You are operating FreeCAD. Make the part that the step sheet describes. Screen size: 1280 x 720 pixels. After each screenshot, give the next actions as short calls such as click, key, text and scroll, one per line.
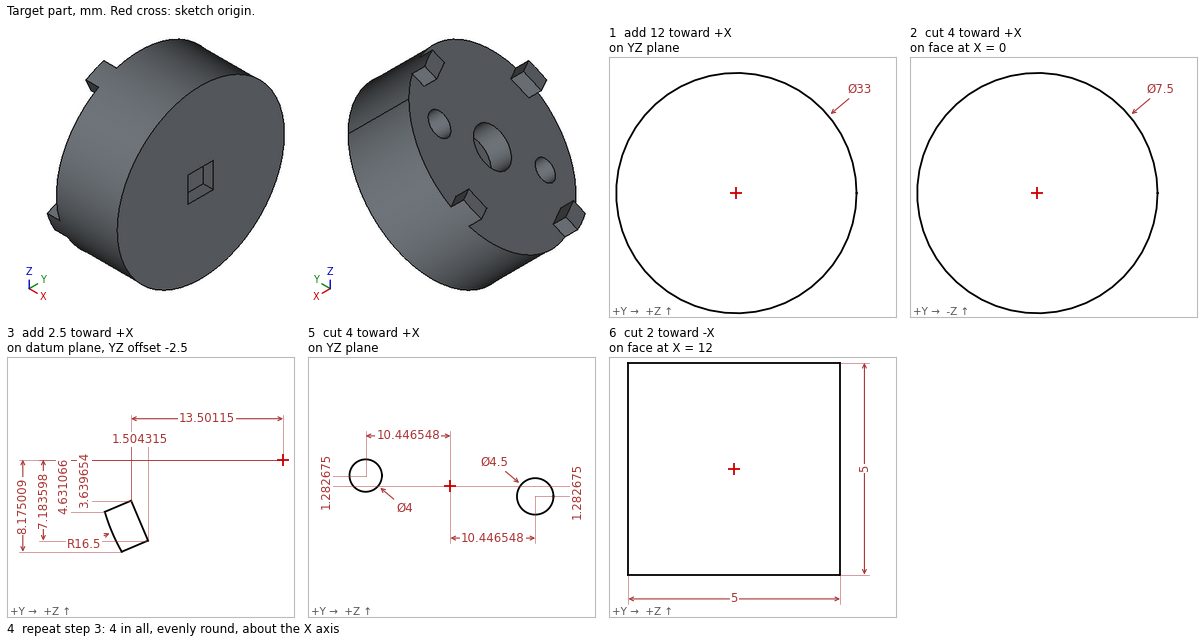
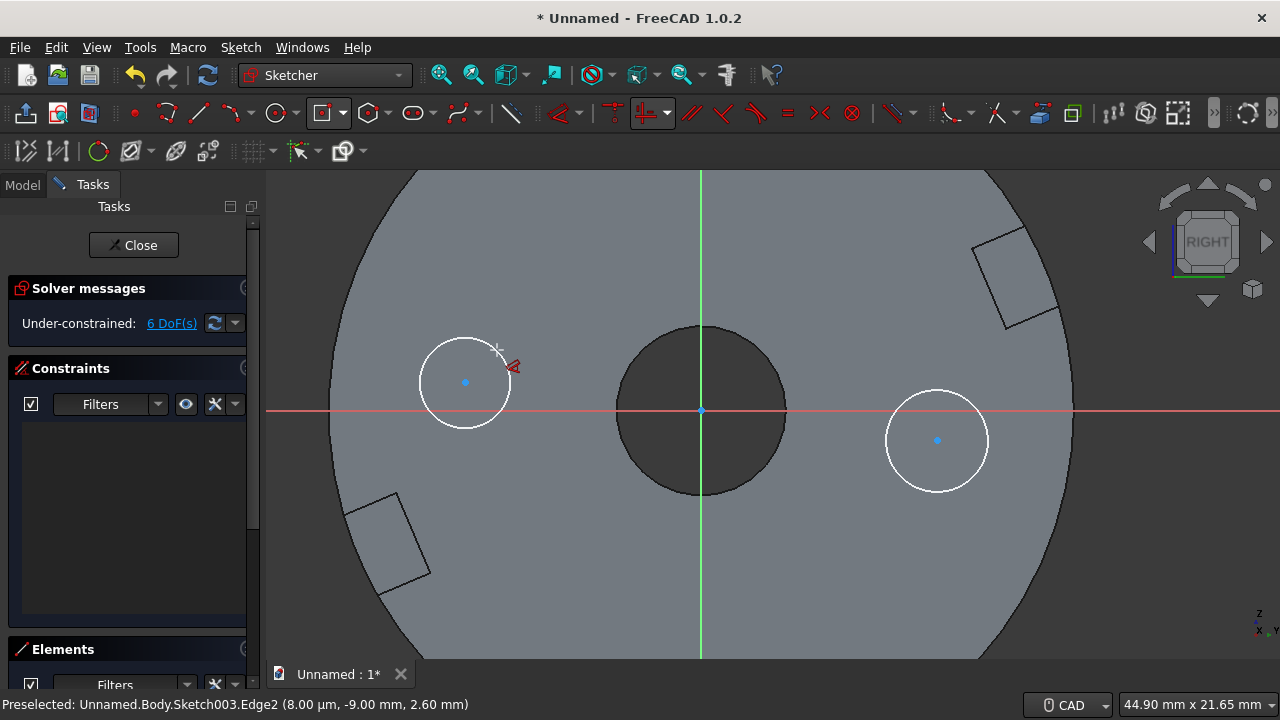
click(901, 477)
click(878, 500)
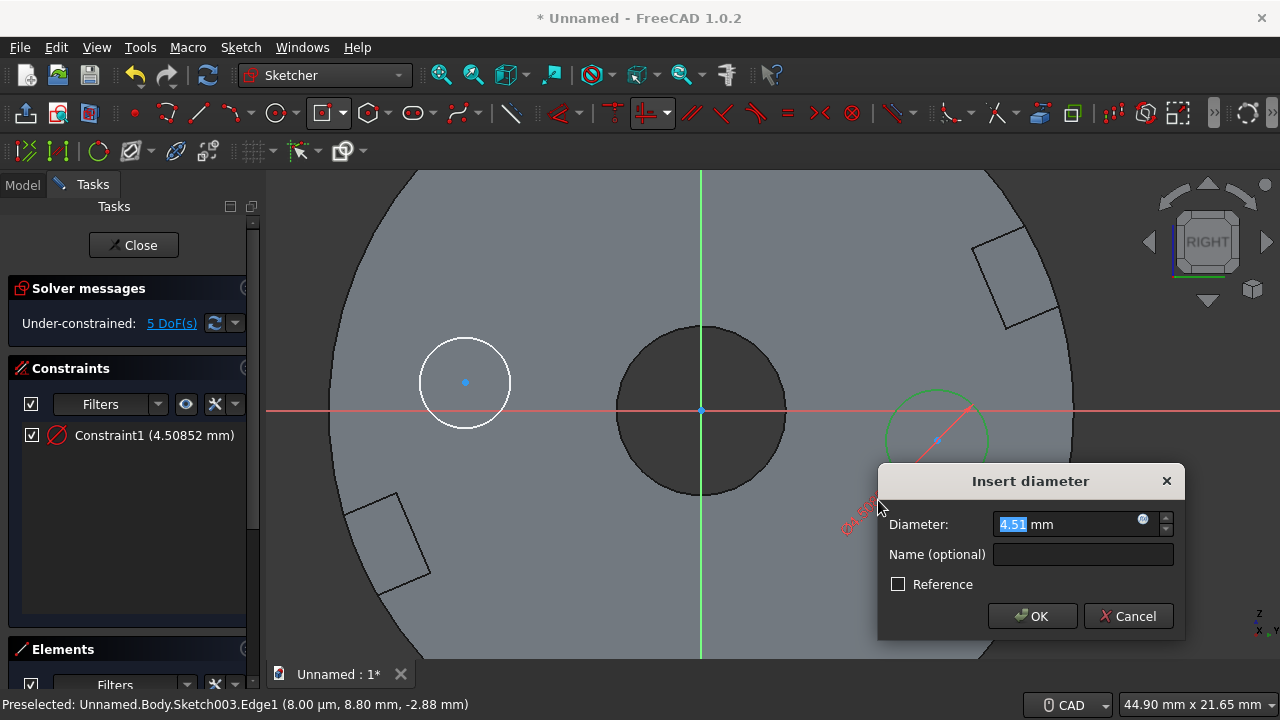
text(4.5)
key(Return)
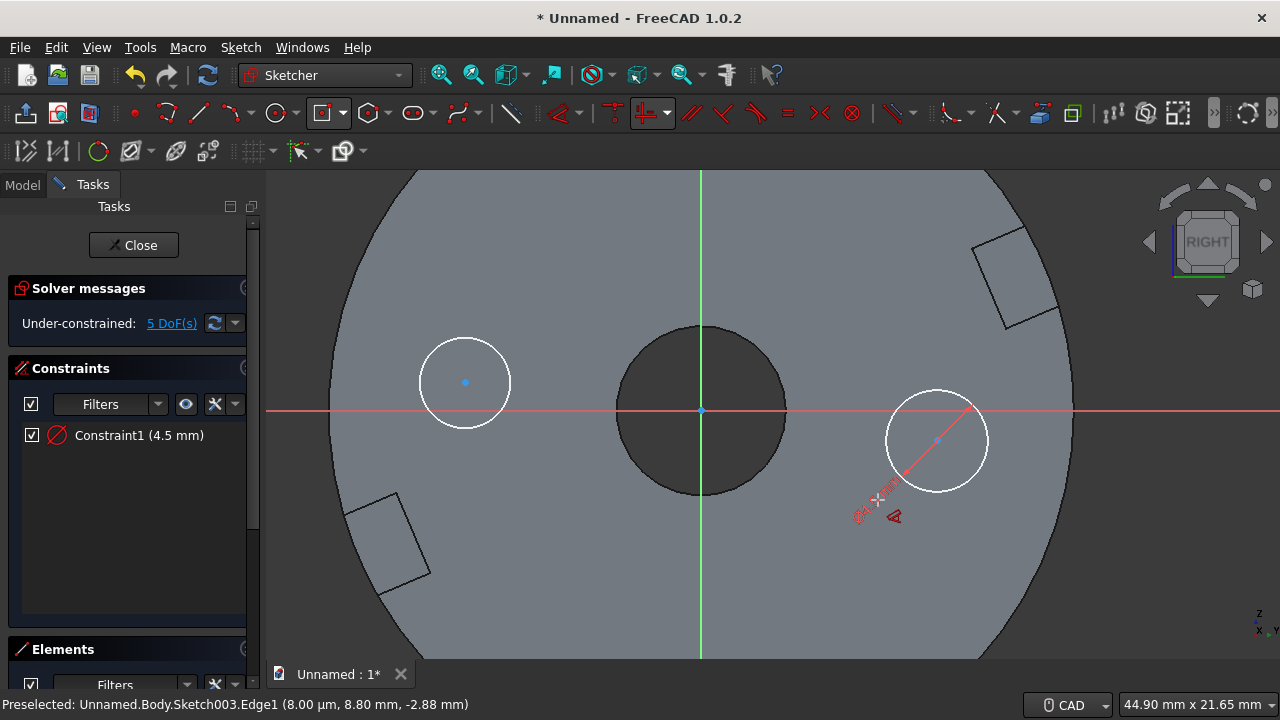
click(497, 351)
click(520, 328)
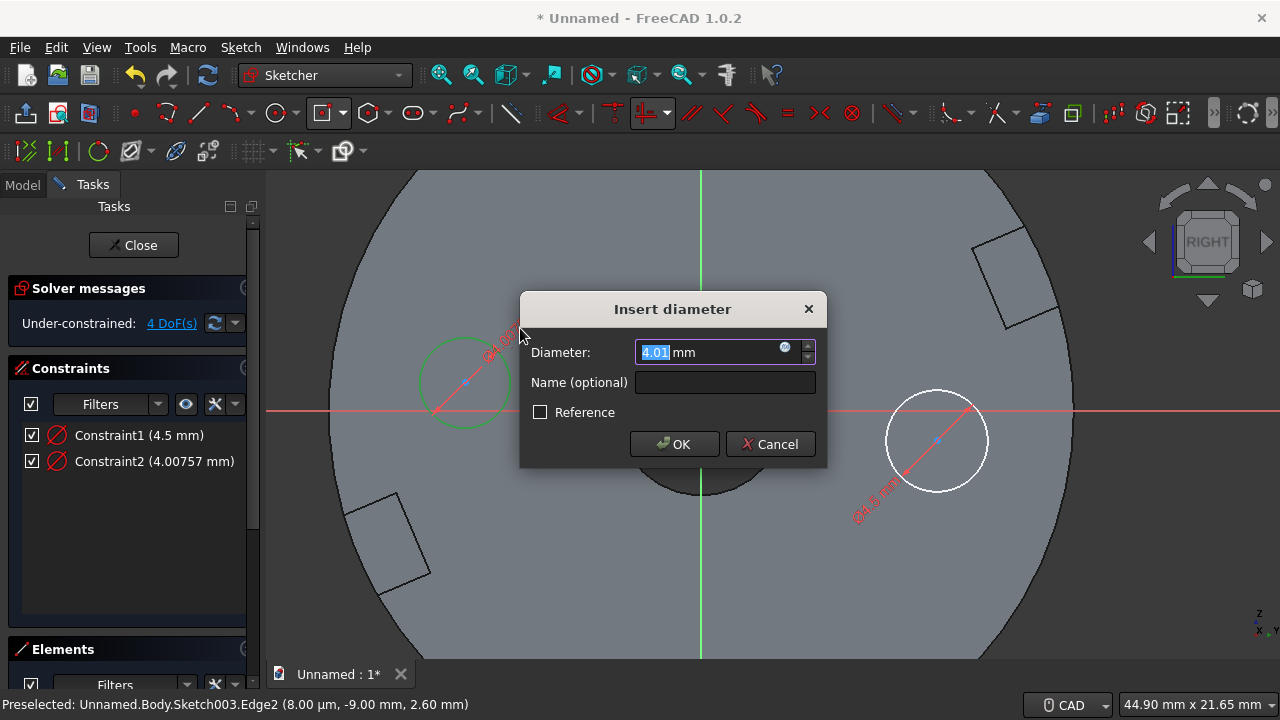
text(4)
key(Return)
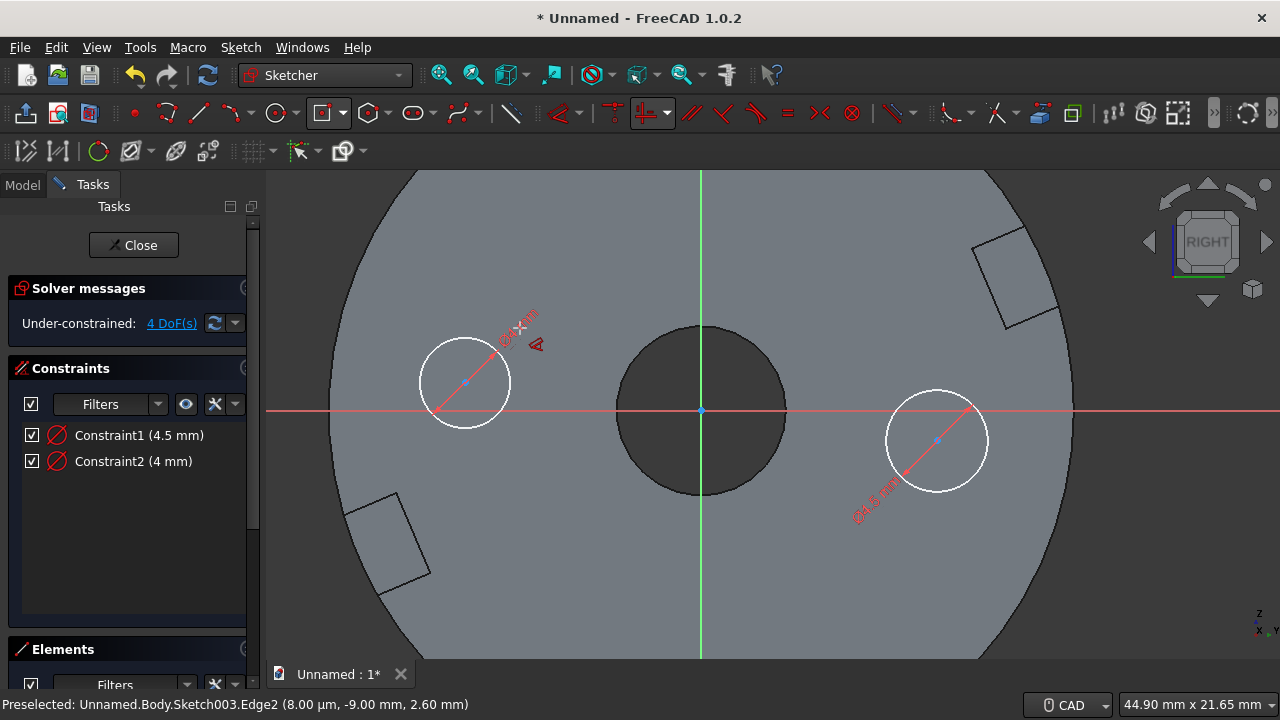
scroll(937, 441, up, 2)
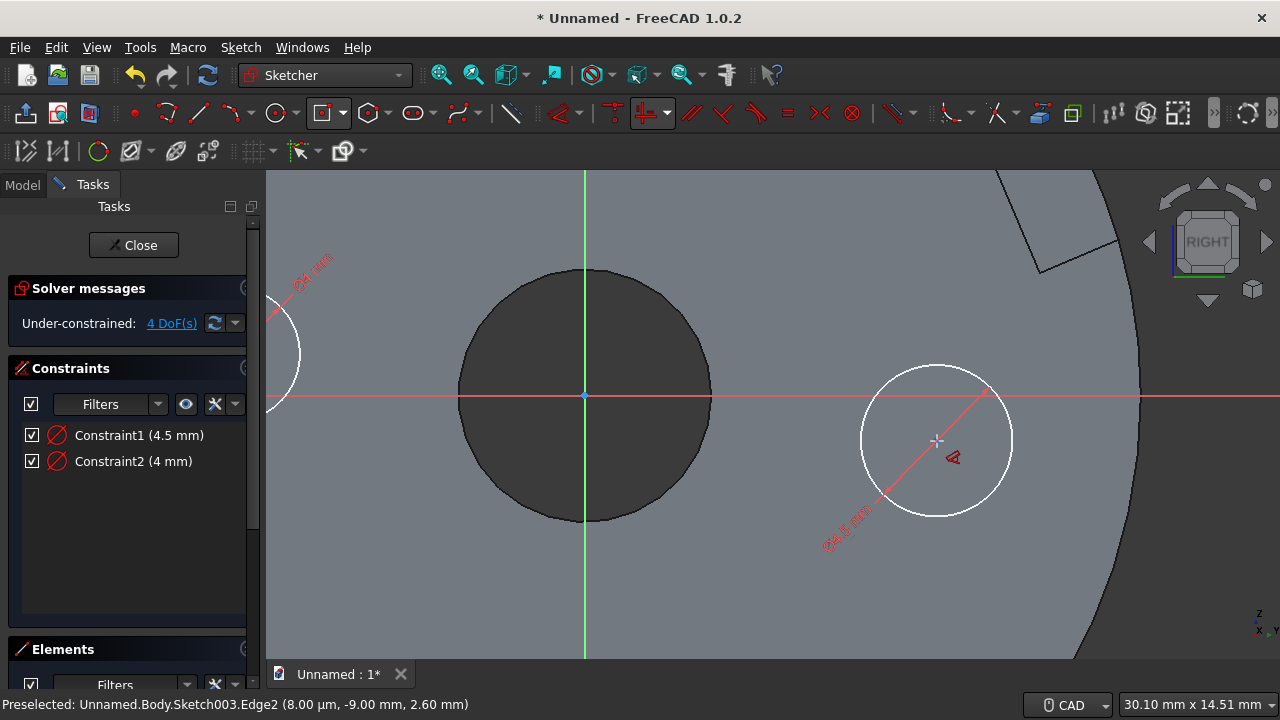
click(937, 441)
click(971, 418)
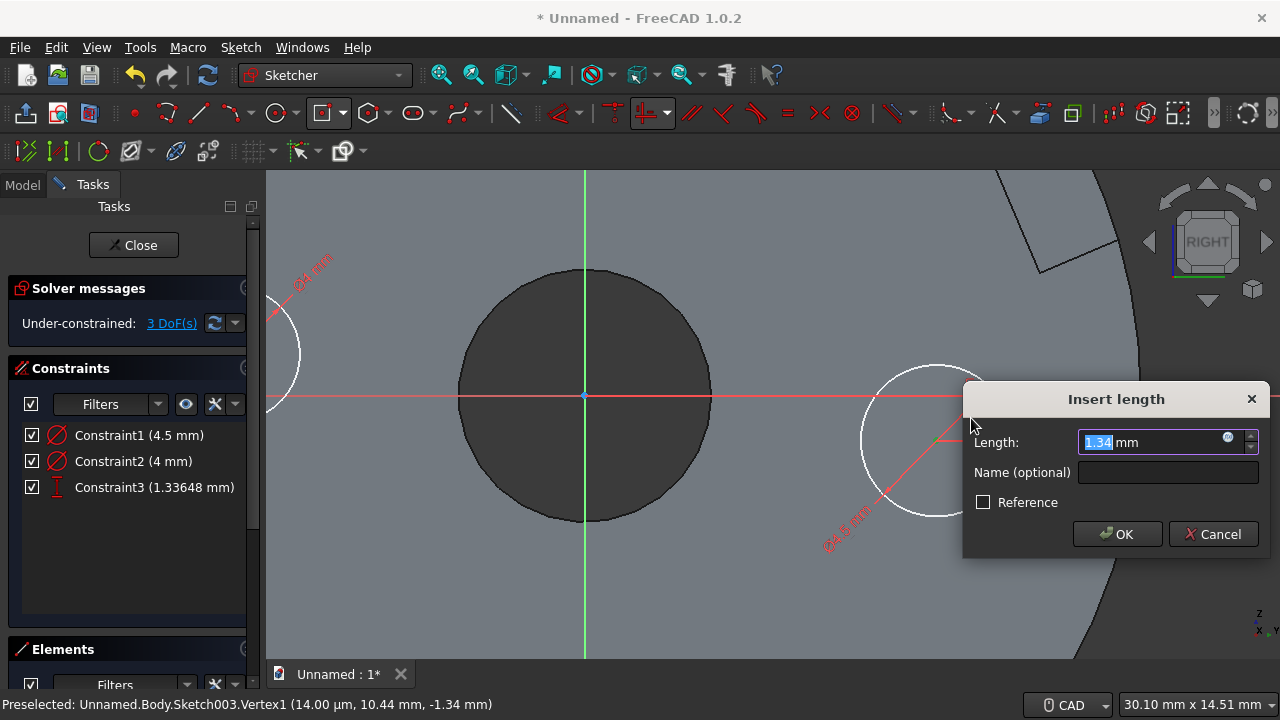
text(1.282675)
key(Return)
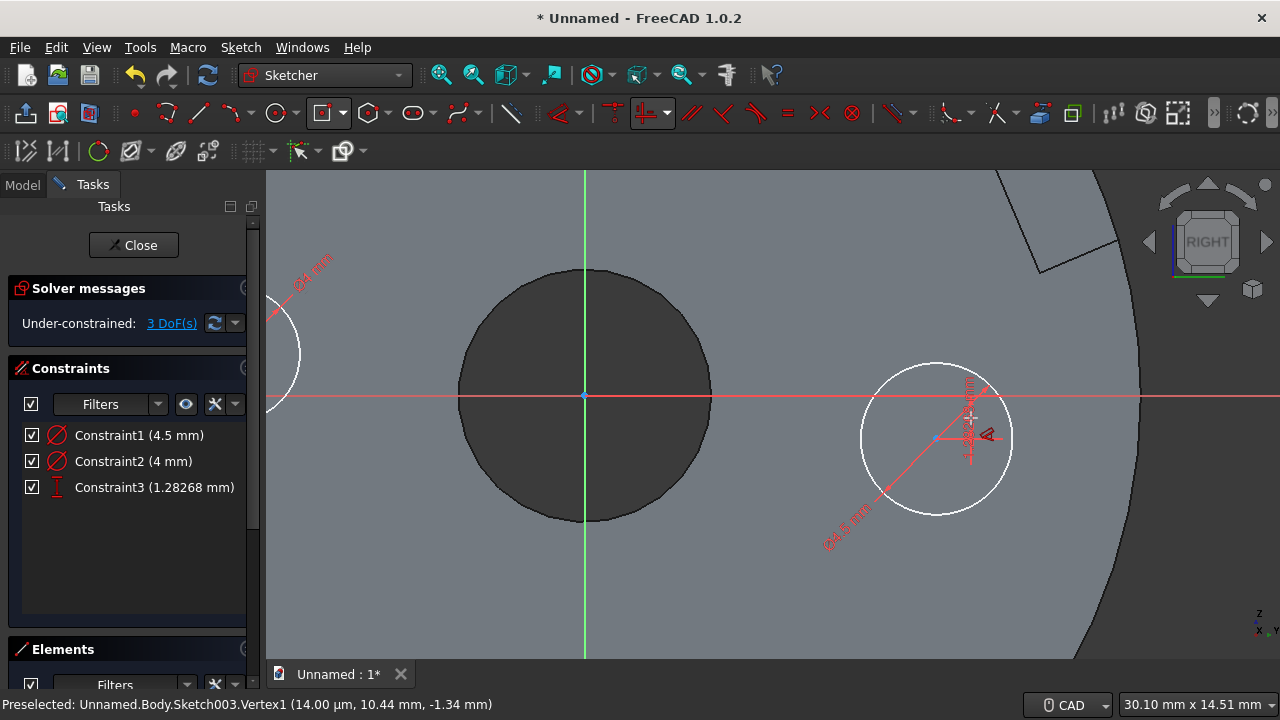
scroll(939, 444, down, 2)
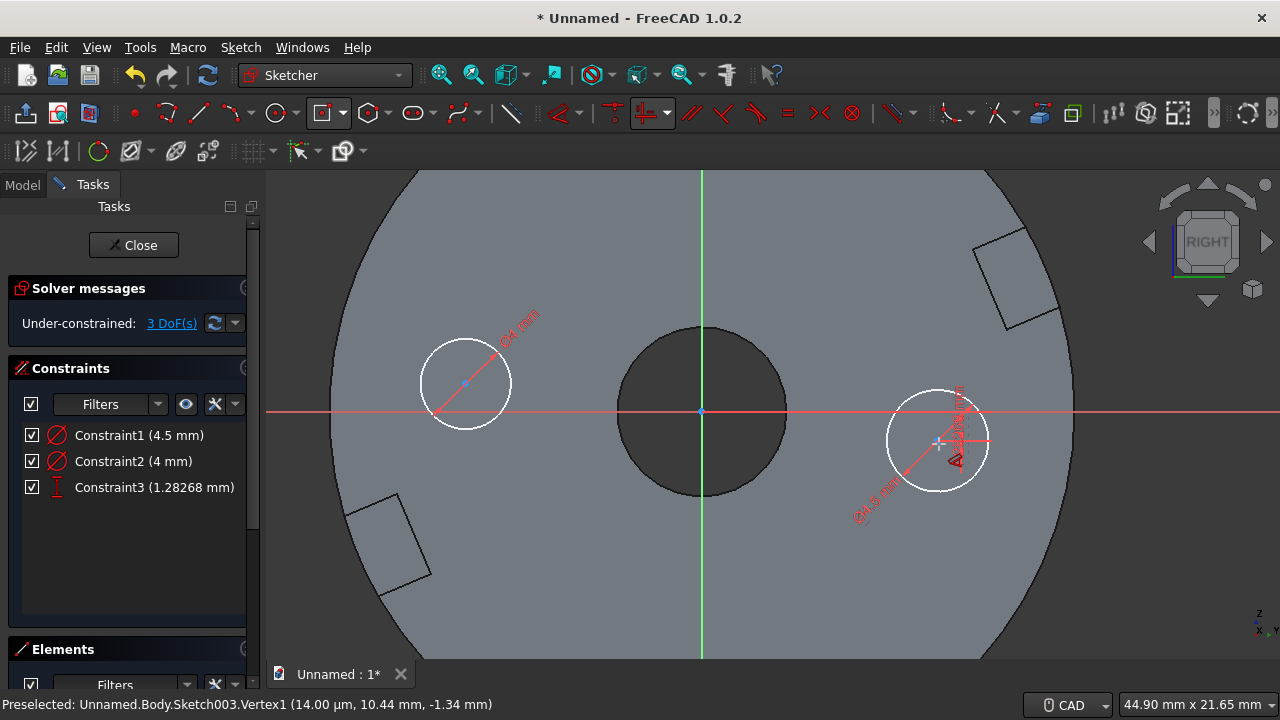
scroll(466, 384, up, 2)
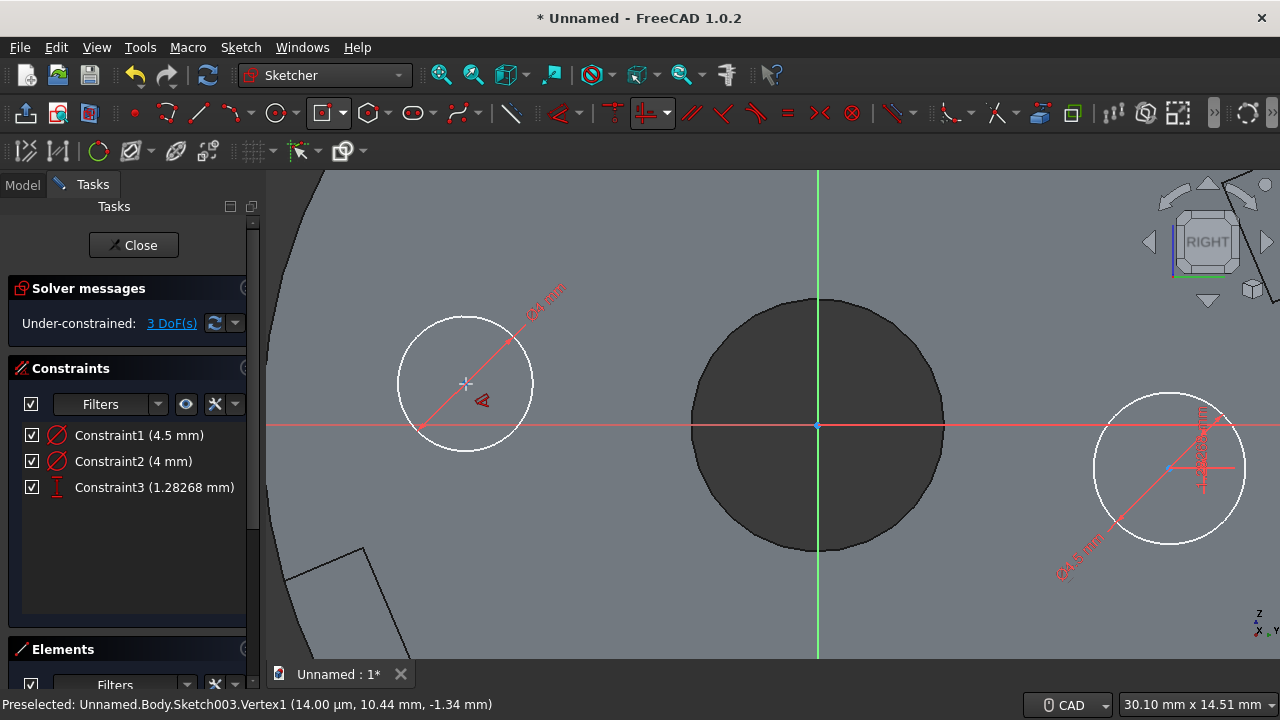
click(465, 384)
click(431, 405)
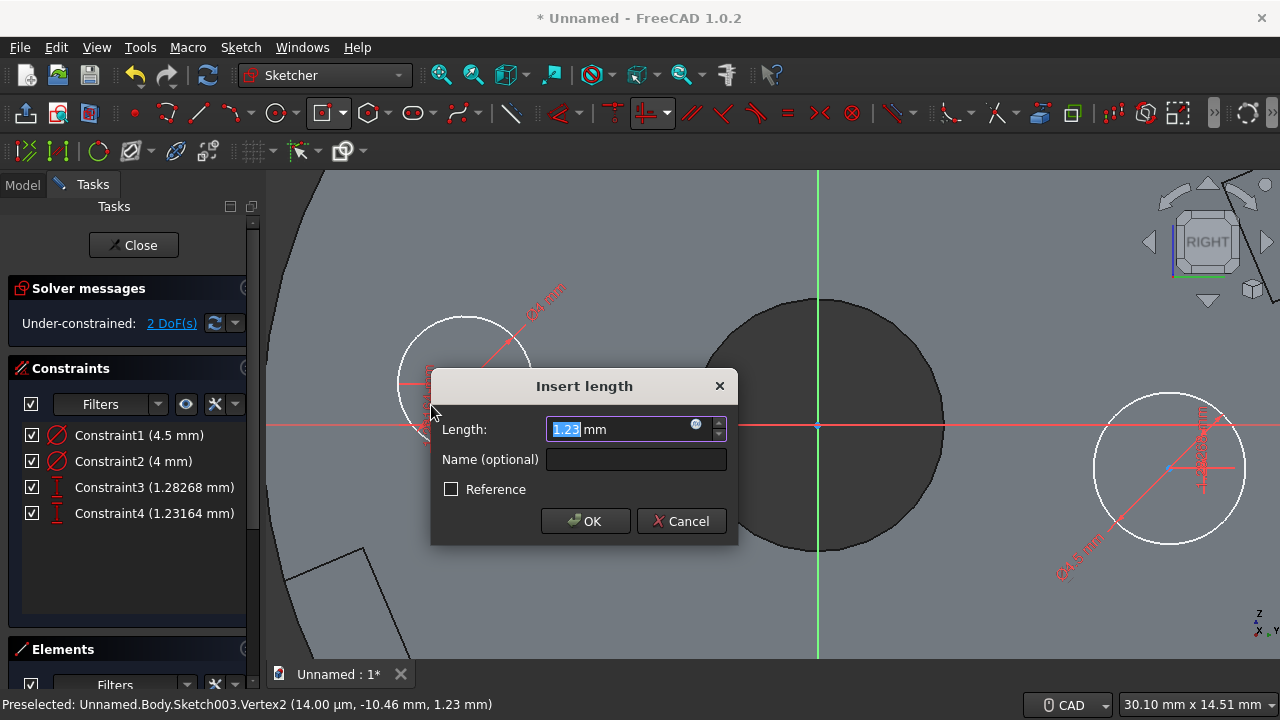
text(1.282675)
key(Return)